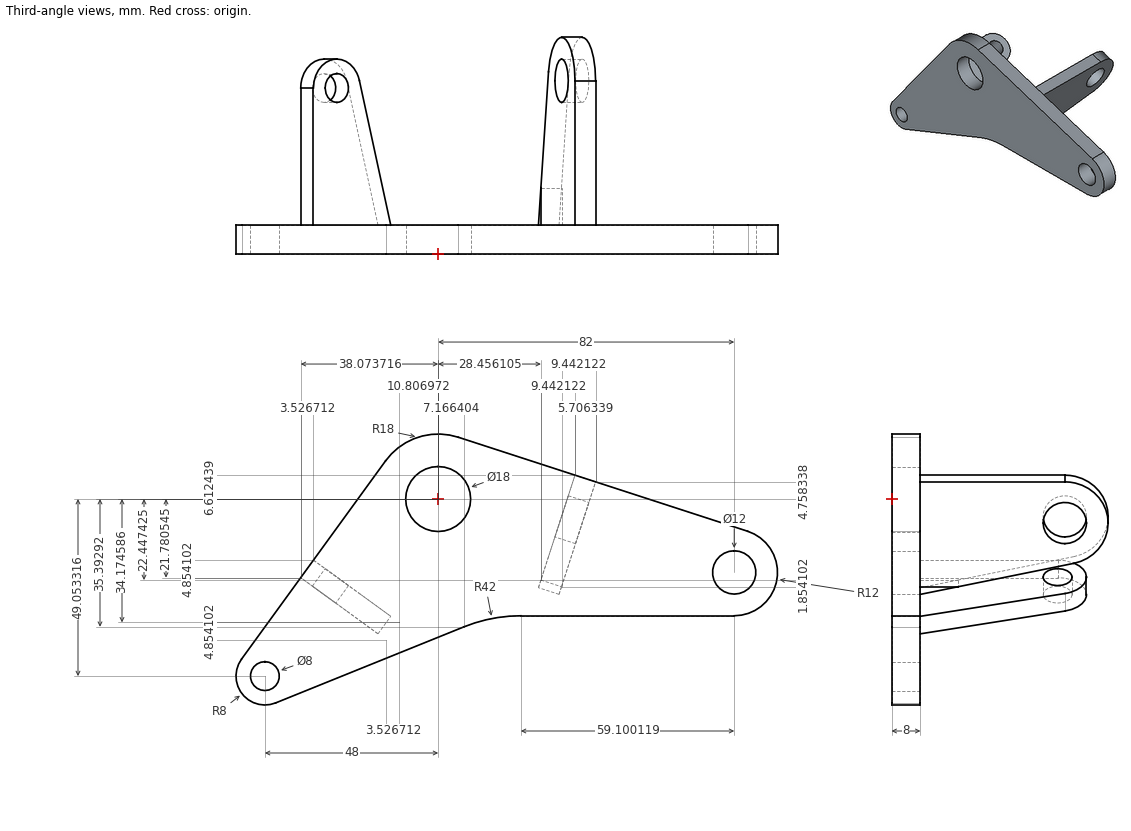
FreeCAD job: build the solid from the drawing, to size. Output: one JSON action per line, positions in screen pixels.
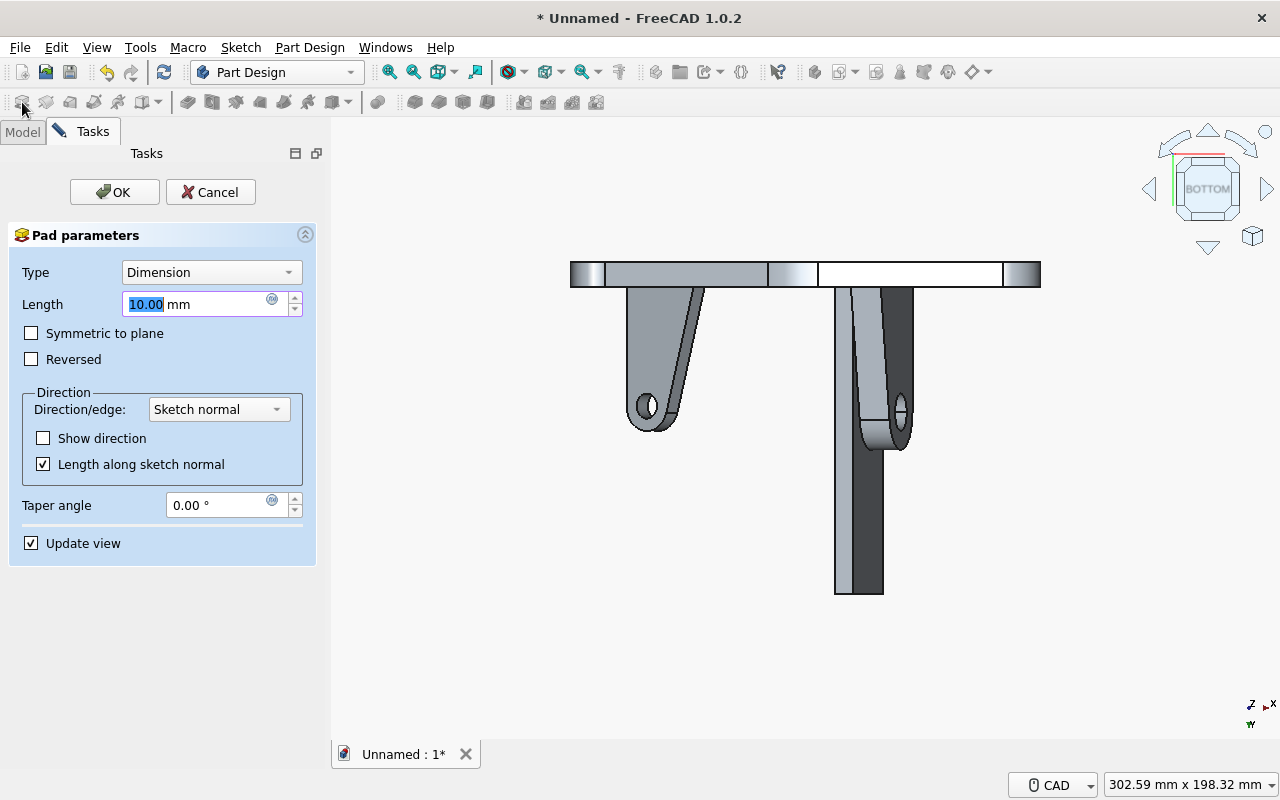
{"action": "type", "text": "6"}
{"action": "key", "text": "Tab"}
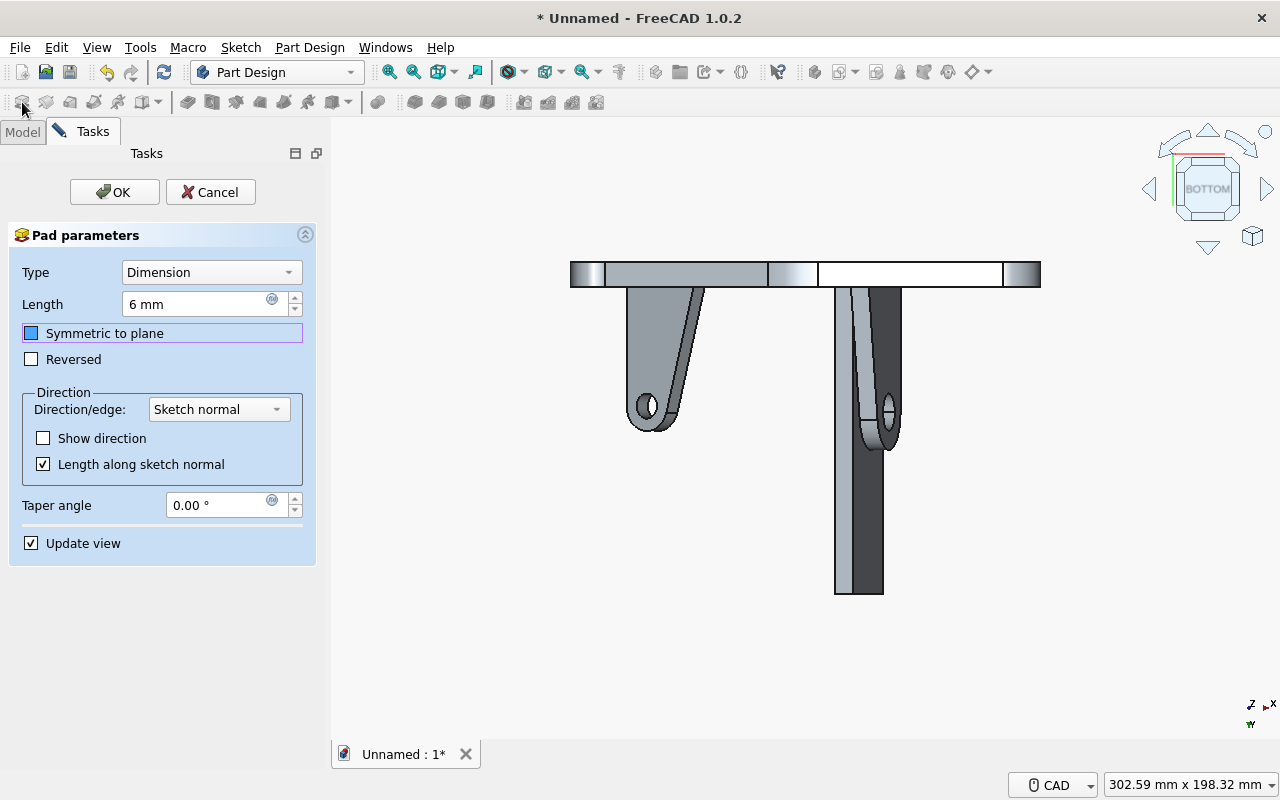
{"action": "left_click", "coordinate": [30, 359]}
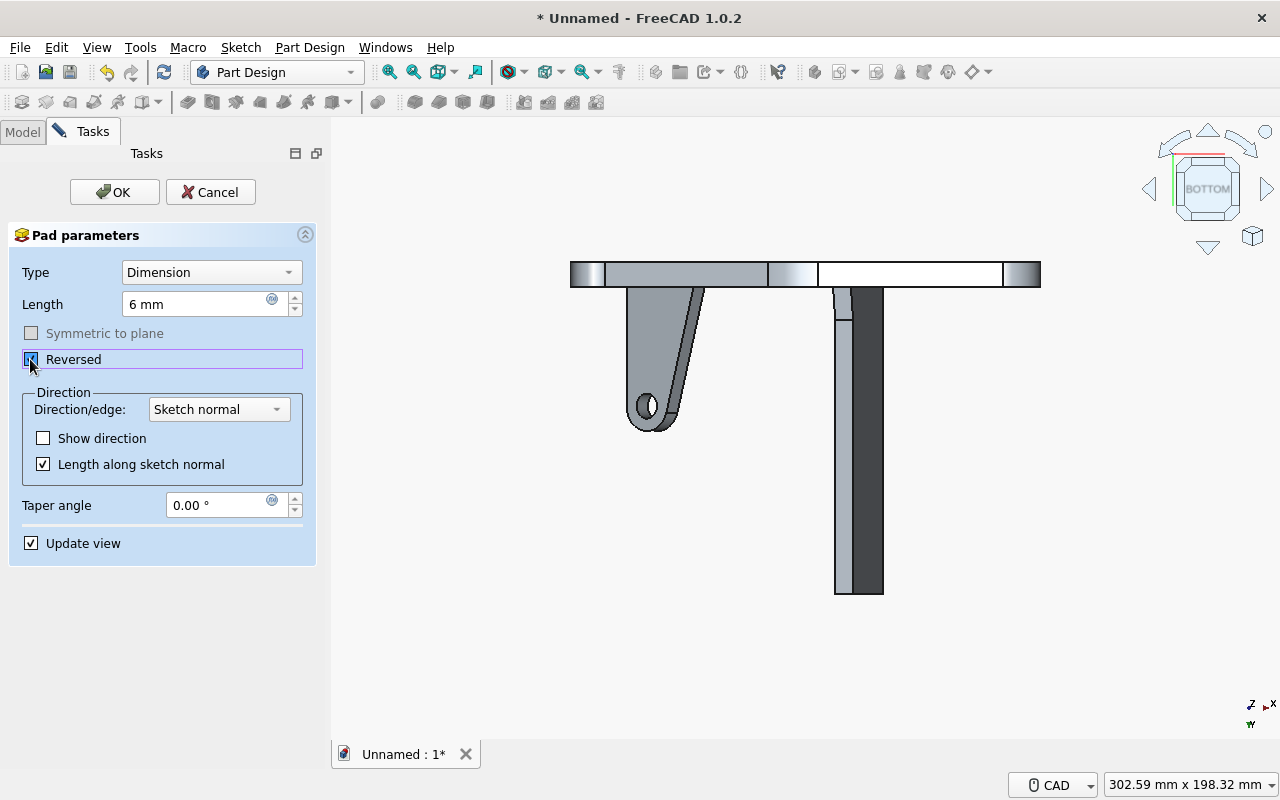
{"action": "left_click", "coordinate": [115, 192]}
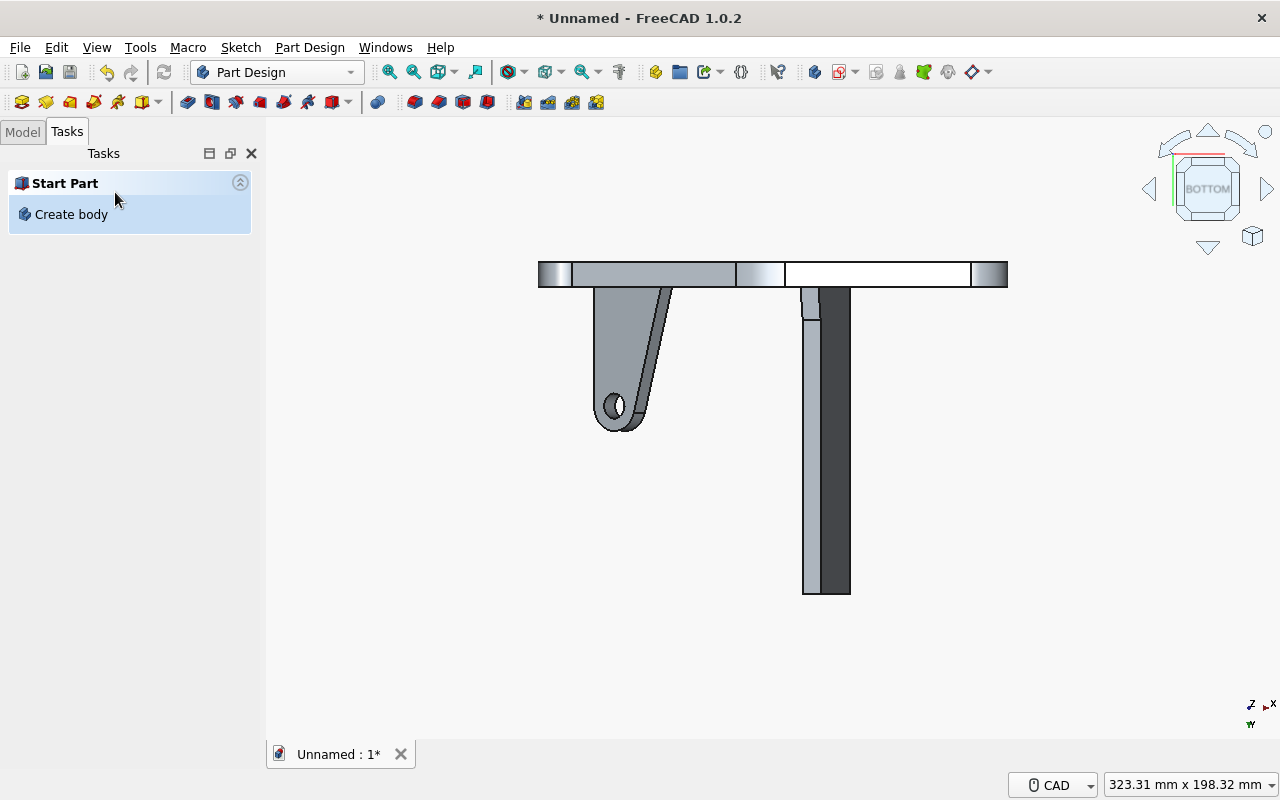
{"action": "left_click", "coordinate": [834, 352]}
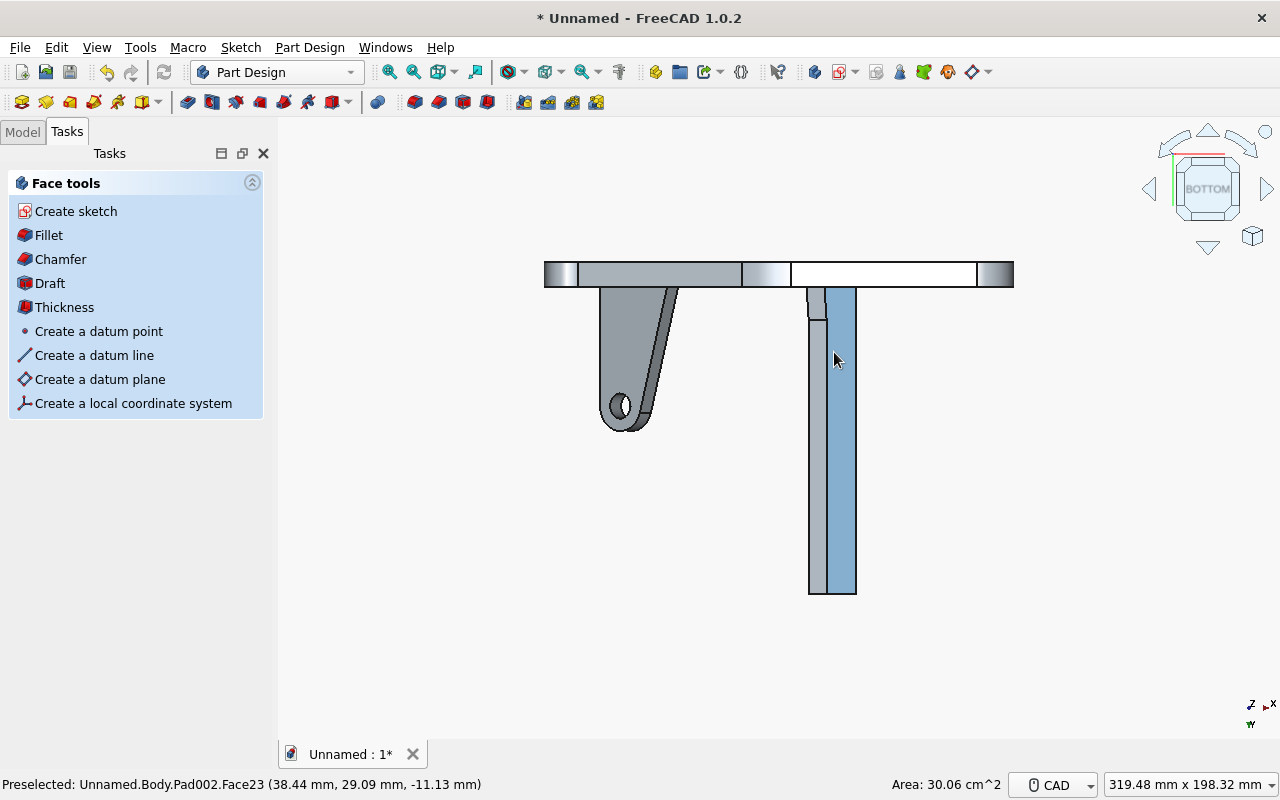
{"action": "left_click", "coordinate": [840, 72]}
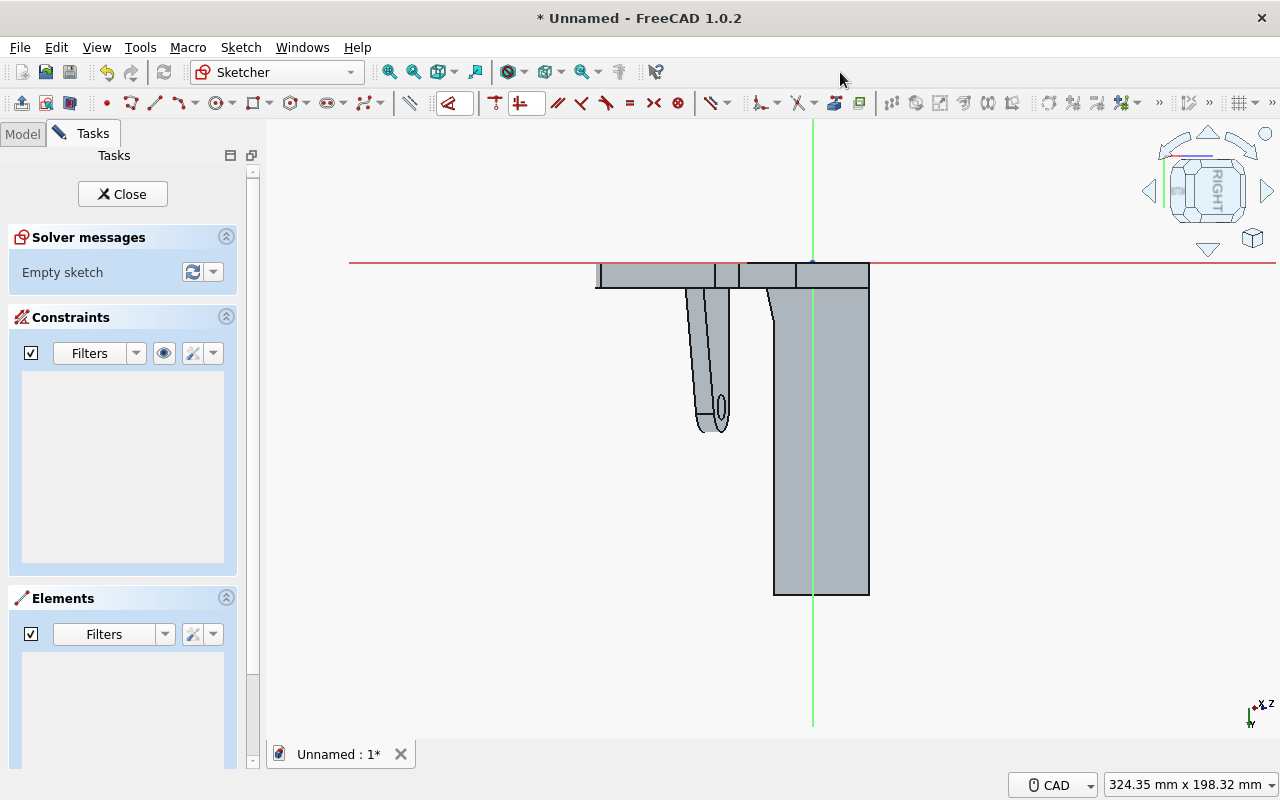
{"action": "key", "text": "g m"}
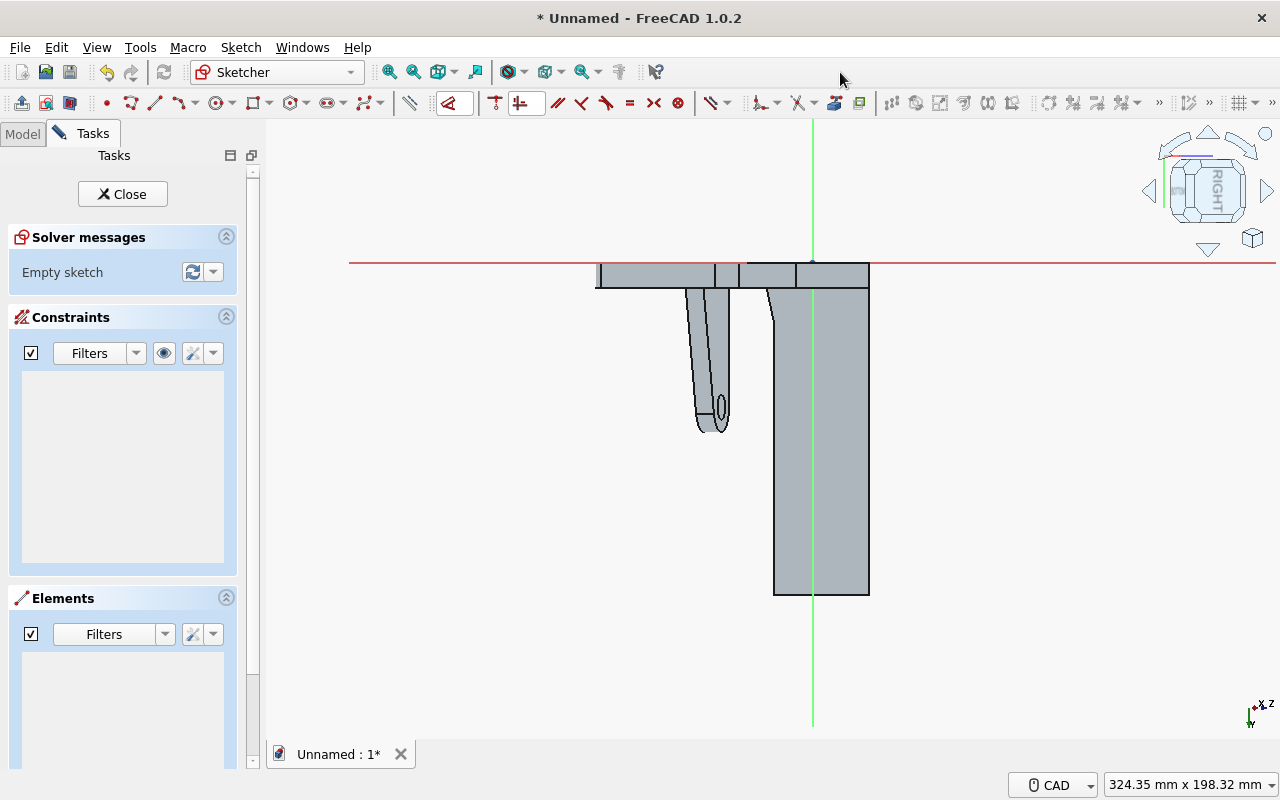
{"action": "left_click", "coordinate": [795, 421]}
{"action": "left_click", "coordinate": [774, 321]}
{"action": "left_click", "coordinate": [711, 621]}
{"action": "left_click", "coordinate": [959, 638]}
{"action": "left_click", "coordinate": [869, 413]}
{"action": "right_click", "coordinate": [869, 413]}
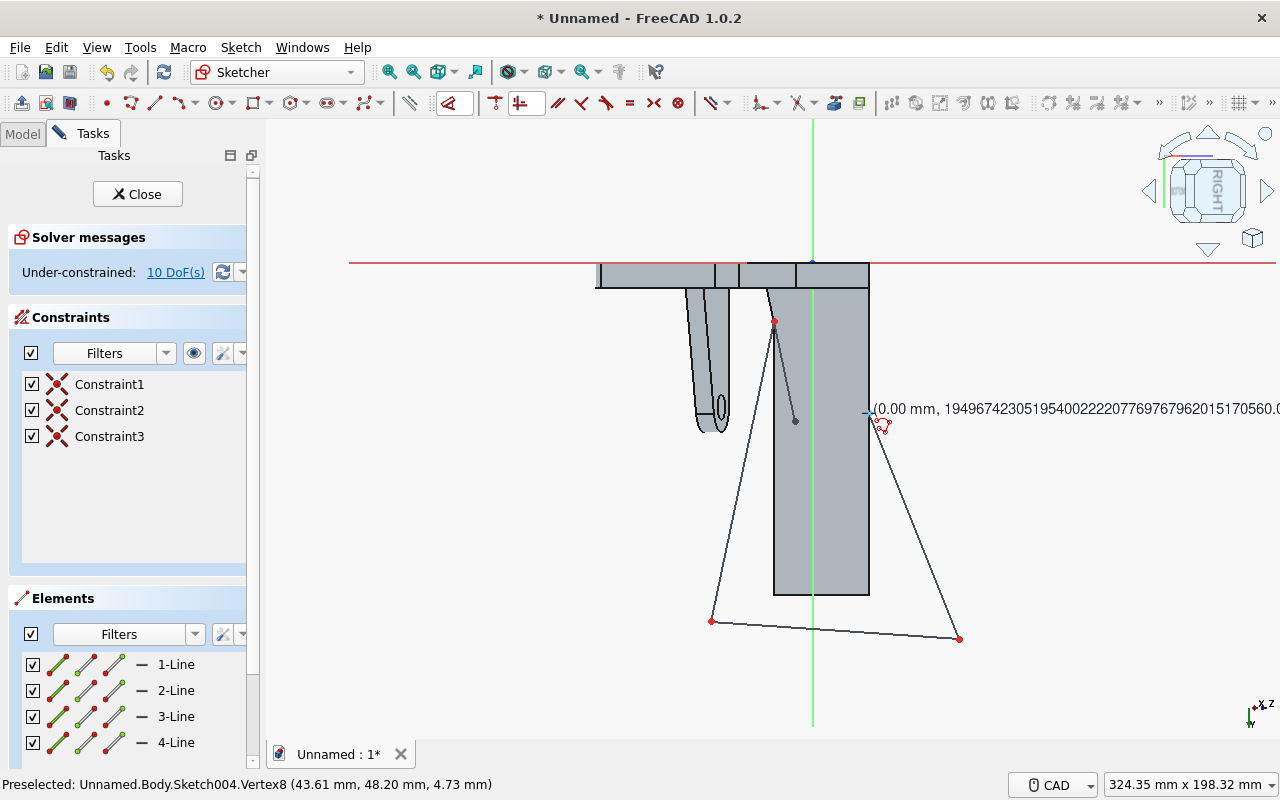
{"action": "key", "text": "g 3 a"}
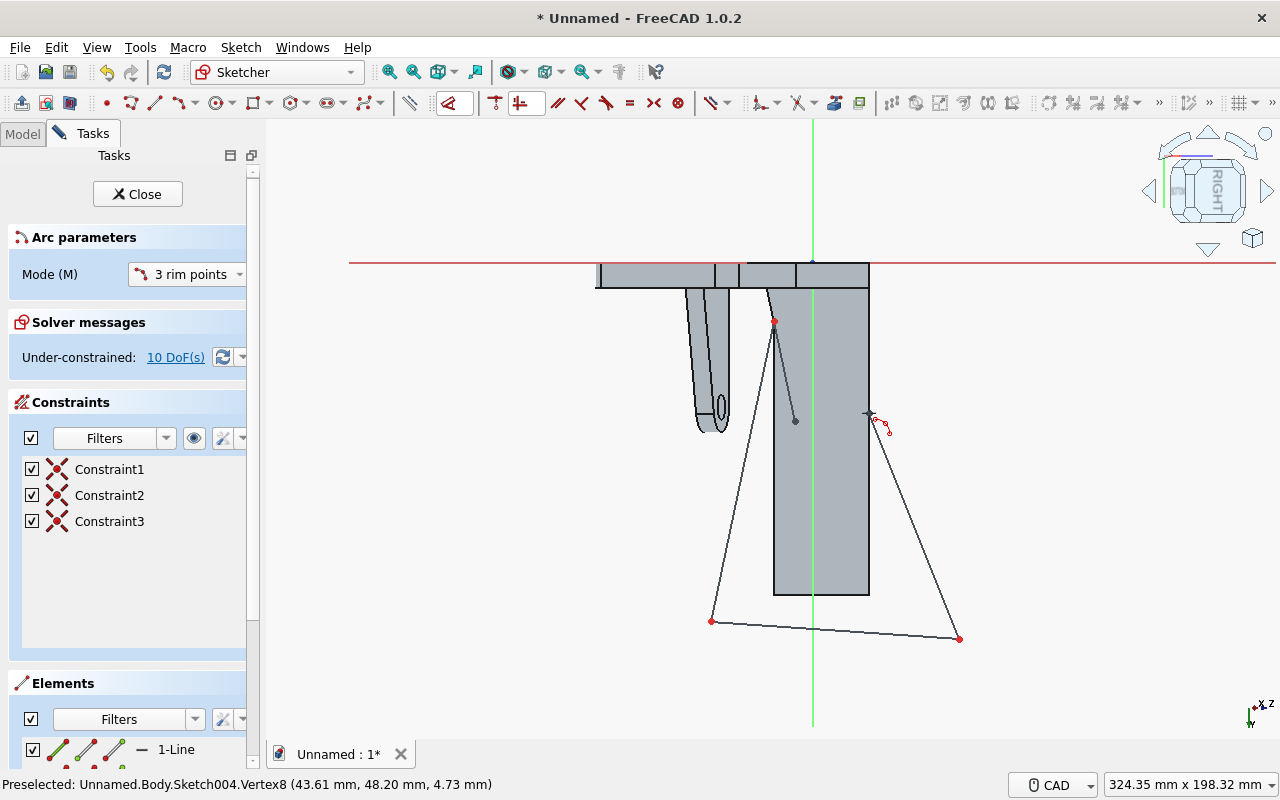
{"action": "left_click", "coordinate": [869, 414]}
{"action": "left_click", "coordinate": [795, 422]}
{"action": "left_click", "coordinate": [835, 451]}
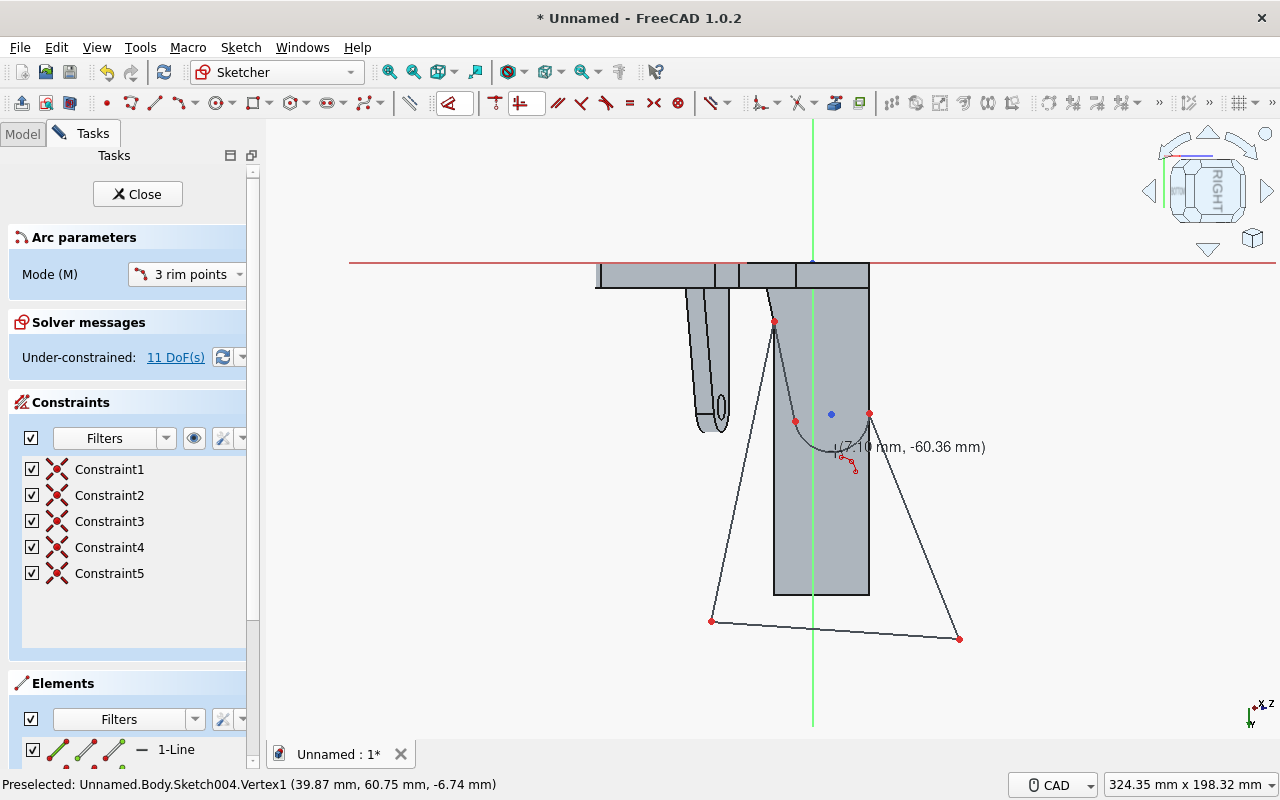
{"action": "left_click", "coordinate": [216, 104]}